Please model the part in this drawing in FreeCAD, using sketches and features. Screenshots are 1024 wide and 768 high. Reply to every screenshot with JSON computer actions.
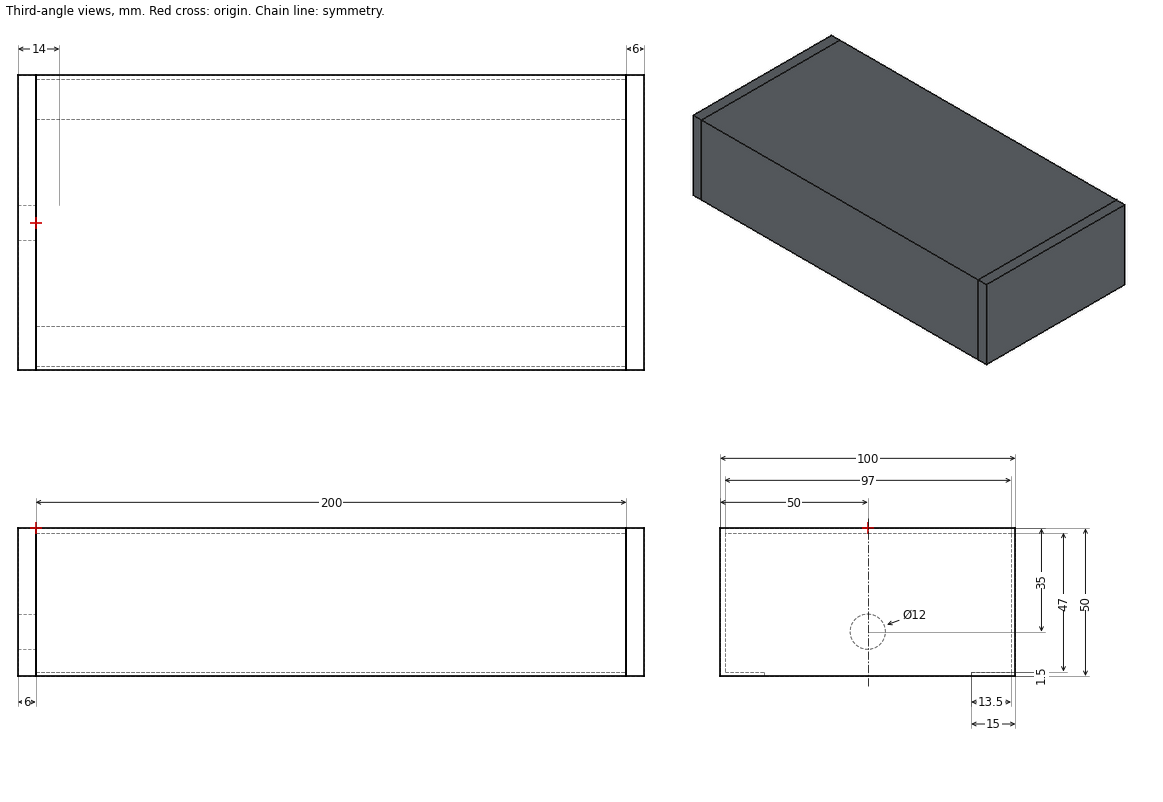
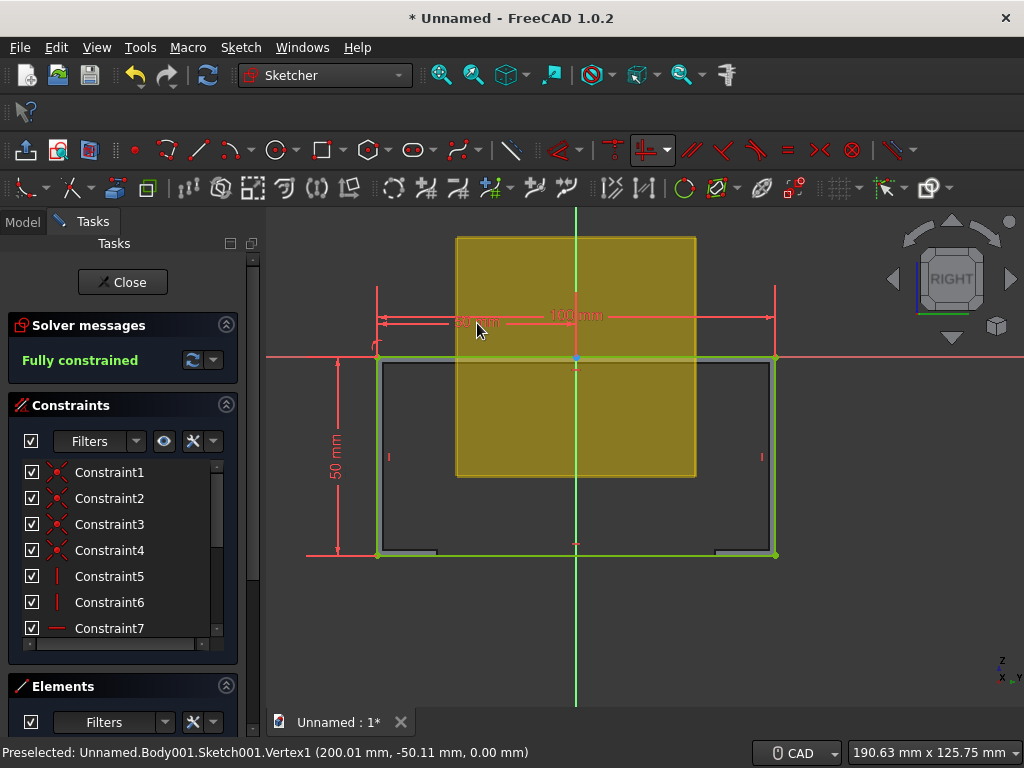
{"action": "left_click", "coordinate": [123, 282]}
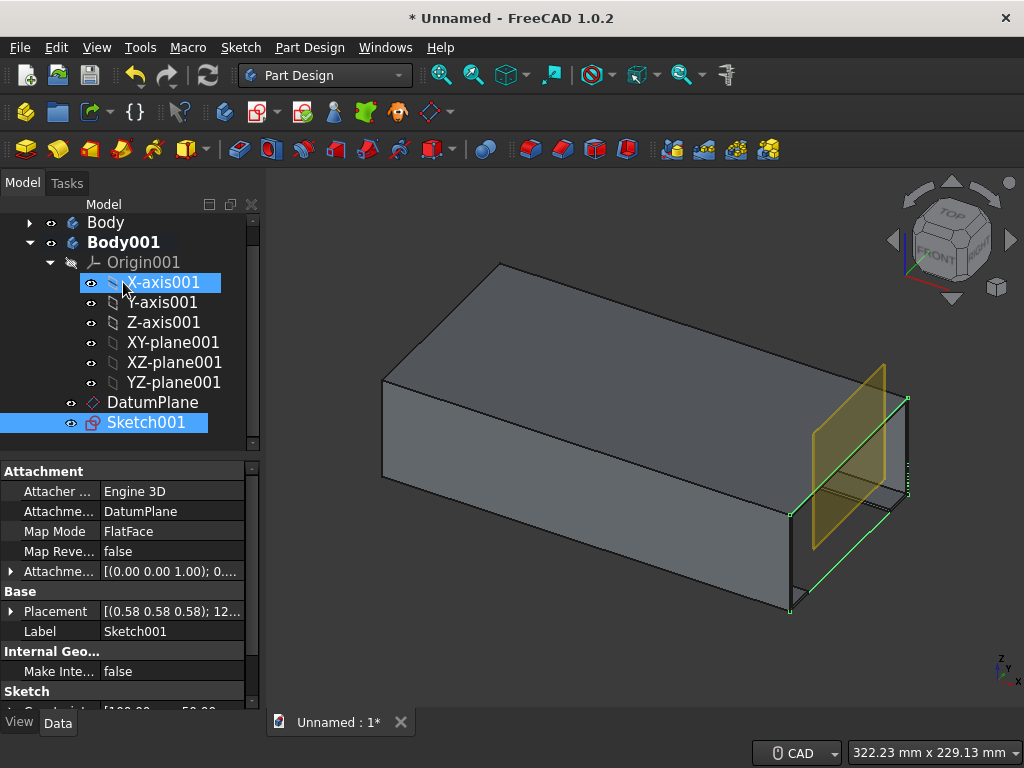
{"action": "left_click", "coordinate": [26, 150]}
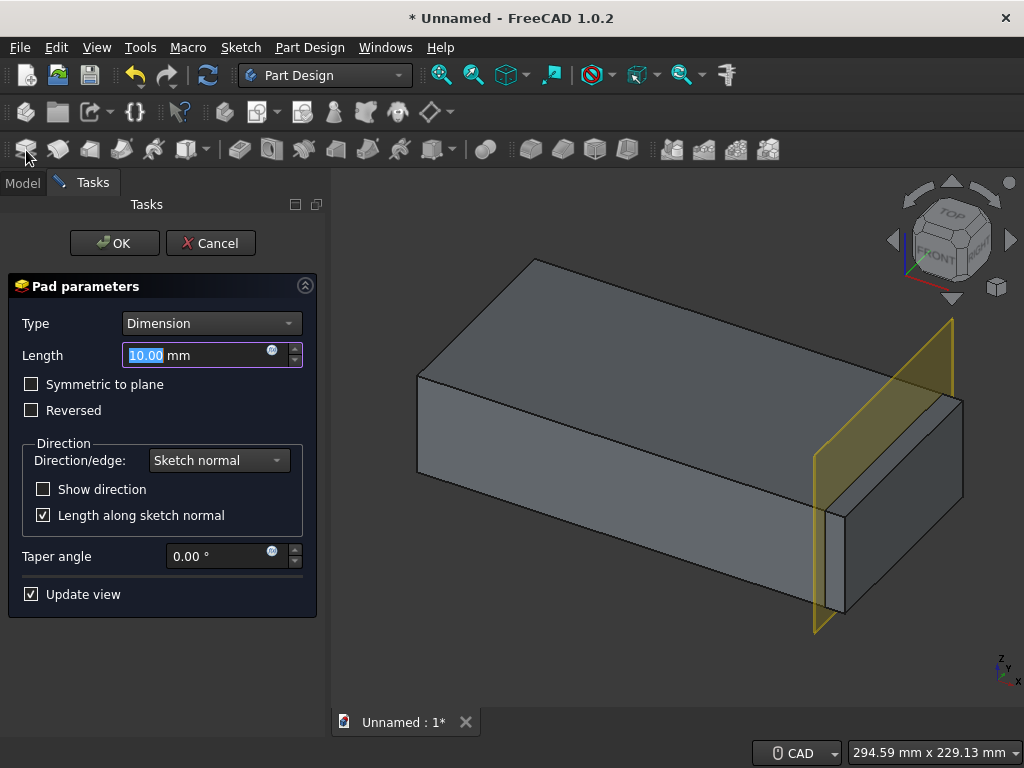
{"action": "type", "text": "6"}
{"action": "key", "text": "Tab"}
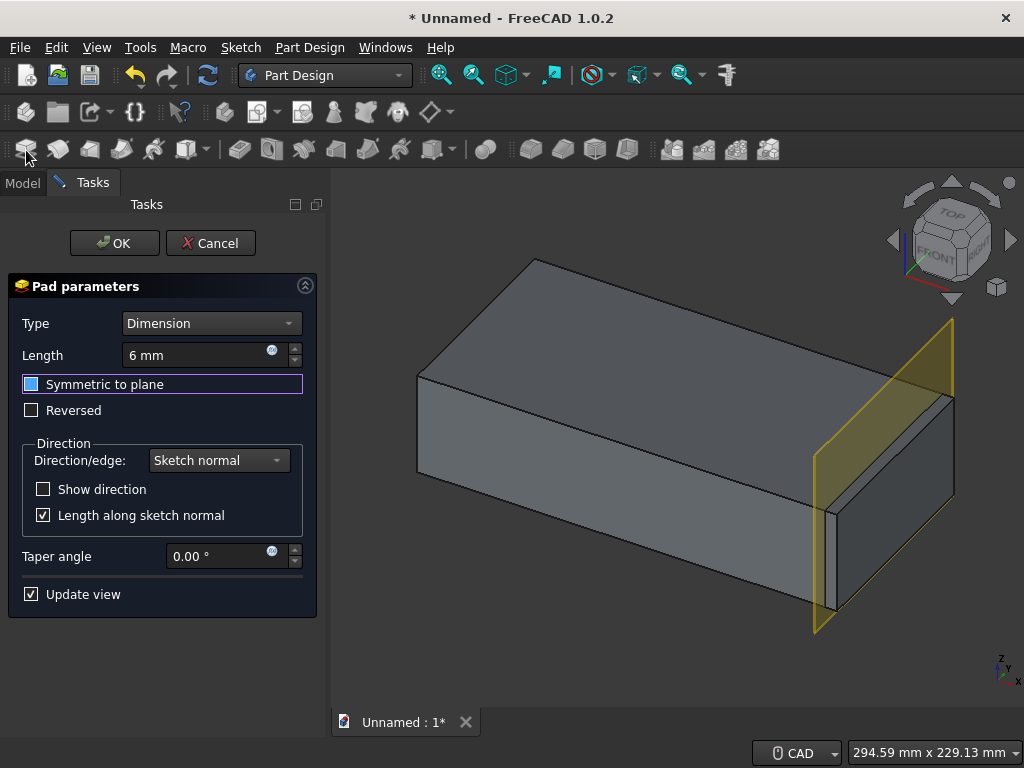
{"action": "left_click", "coordinate": [115, 243]}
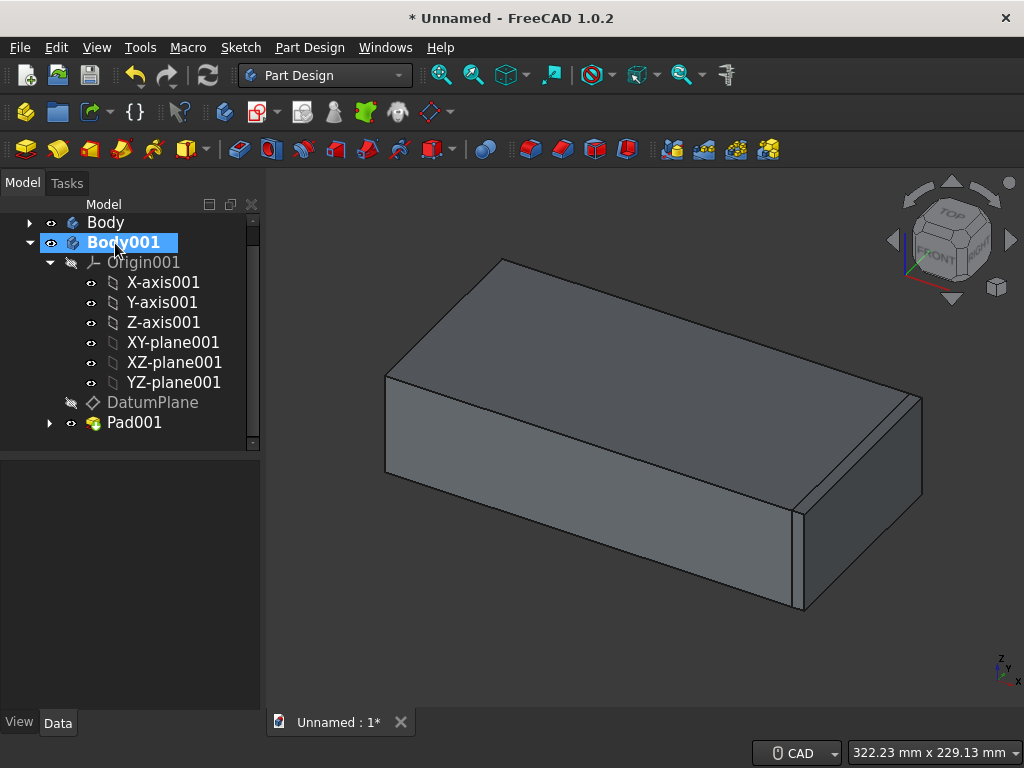
{"action": "left_click", "coordinate": [442, 76]}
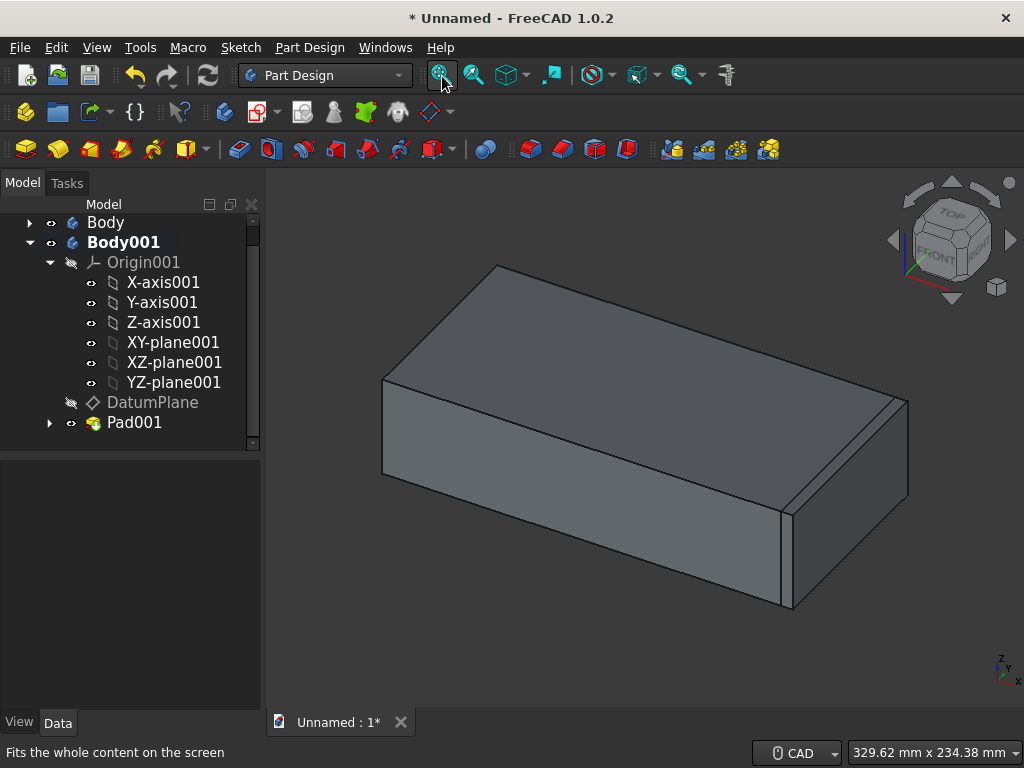
{"action": "left_click", "coordinate": [226, 112]}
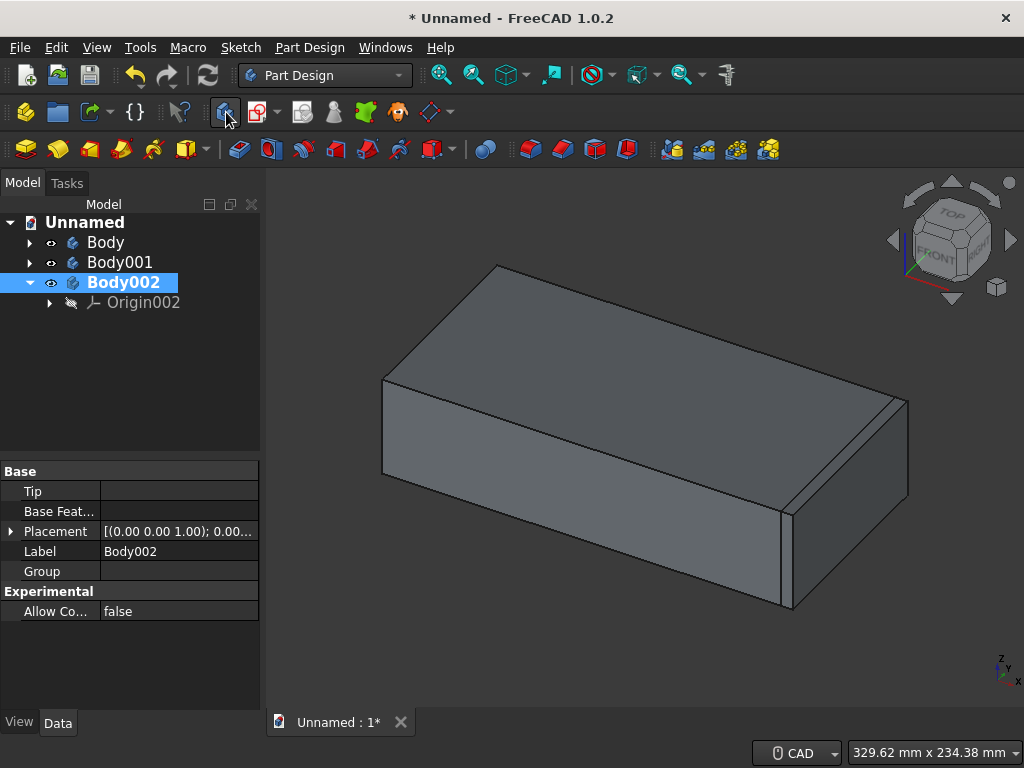
{"action": "left_click", "coordinate": [306, 667]}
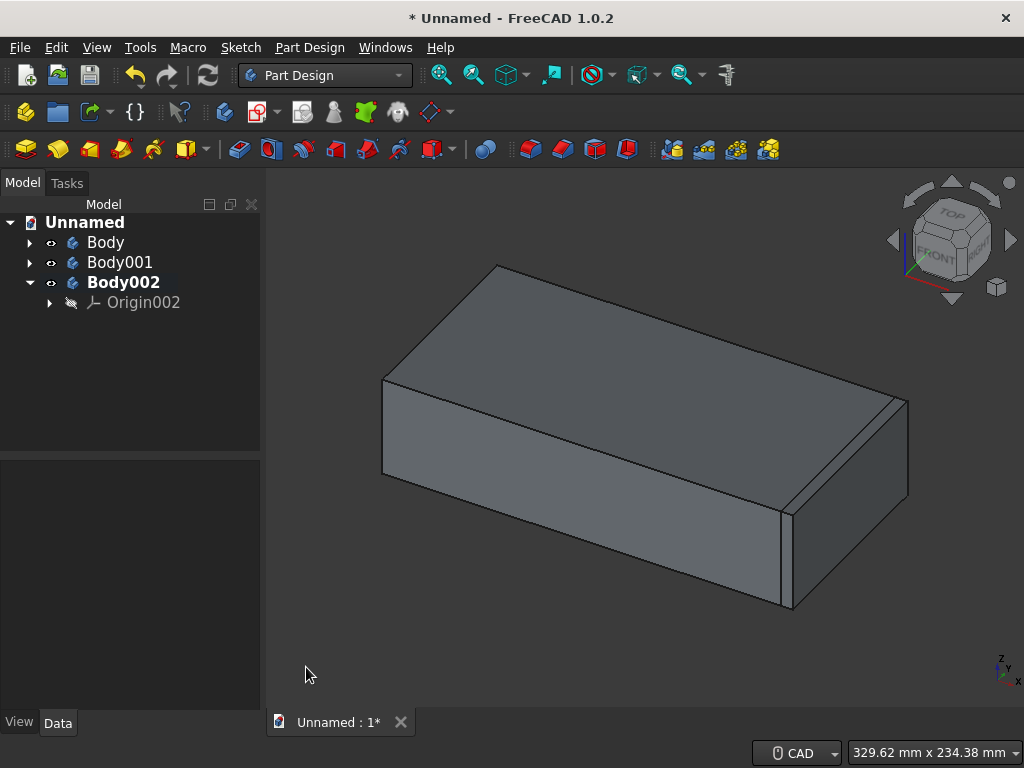
{"action": "left_click", "coordinate": [258, 112]}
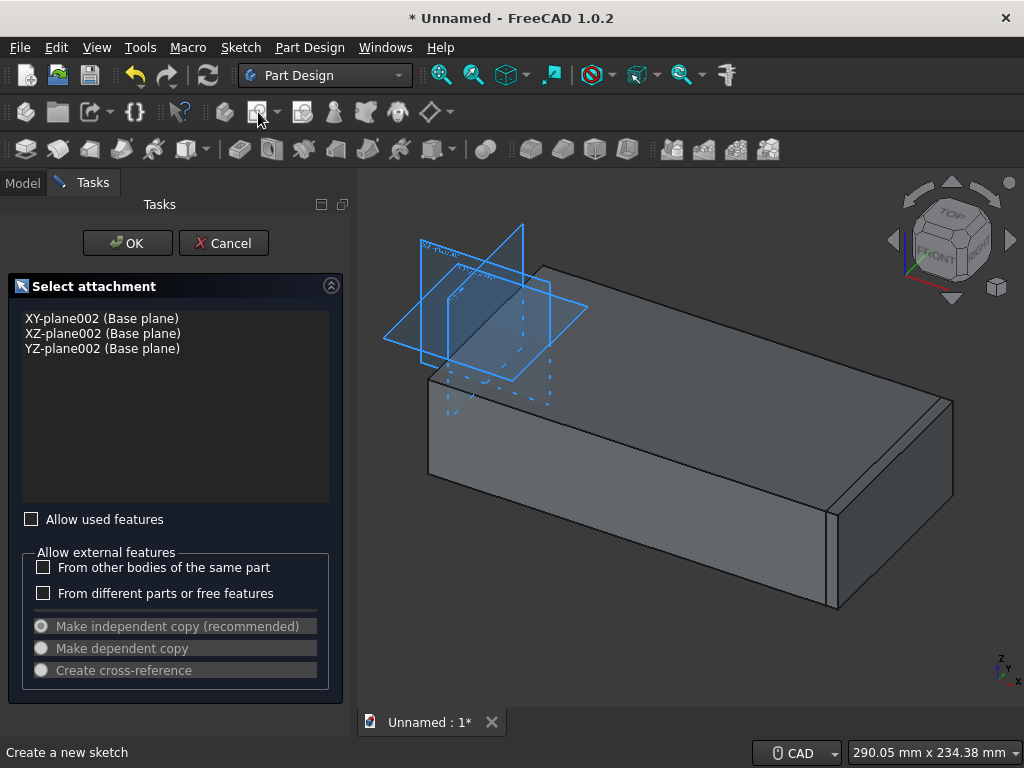
{"action": "left_click", "coordinate": [82, 348]}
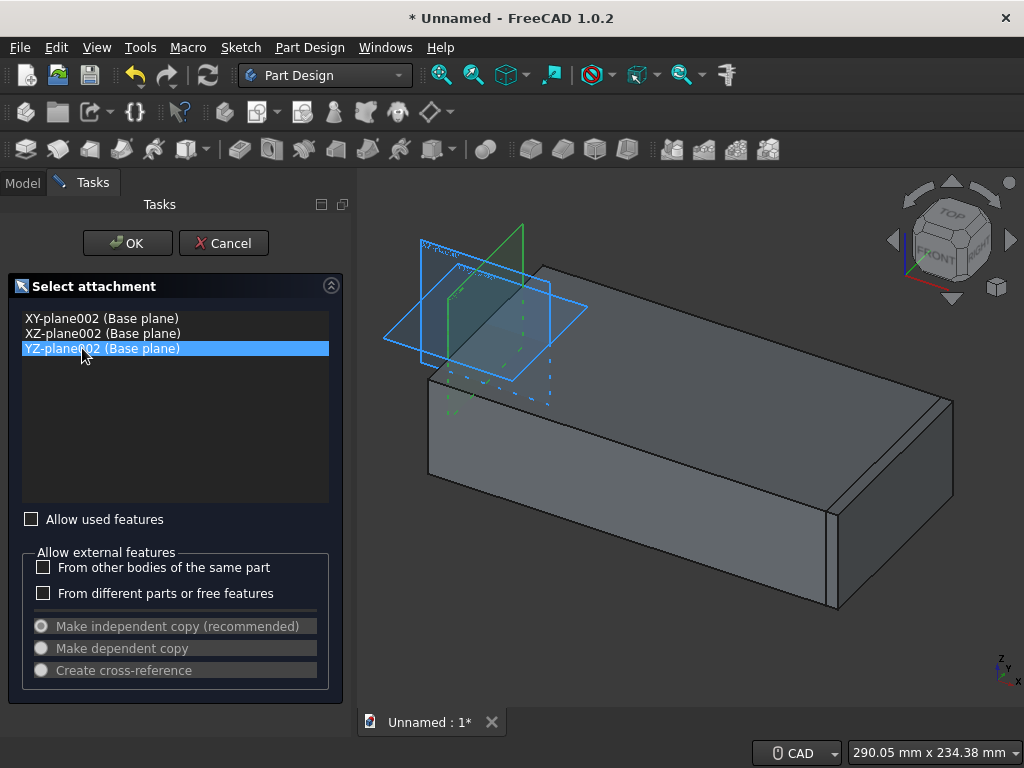
{"action": "left_click", "coordinate": [128, 243]}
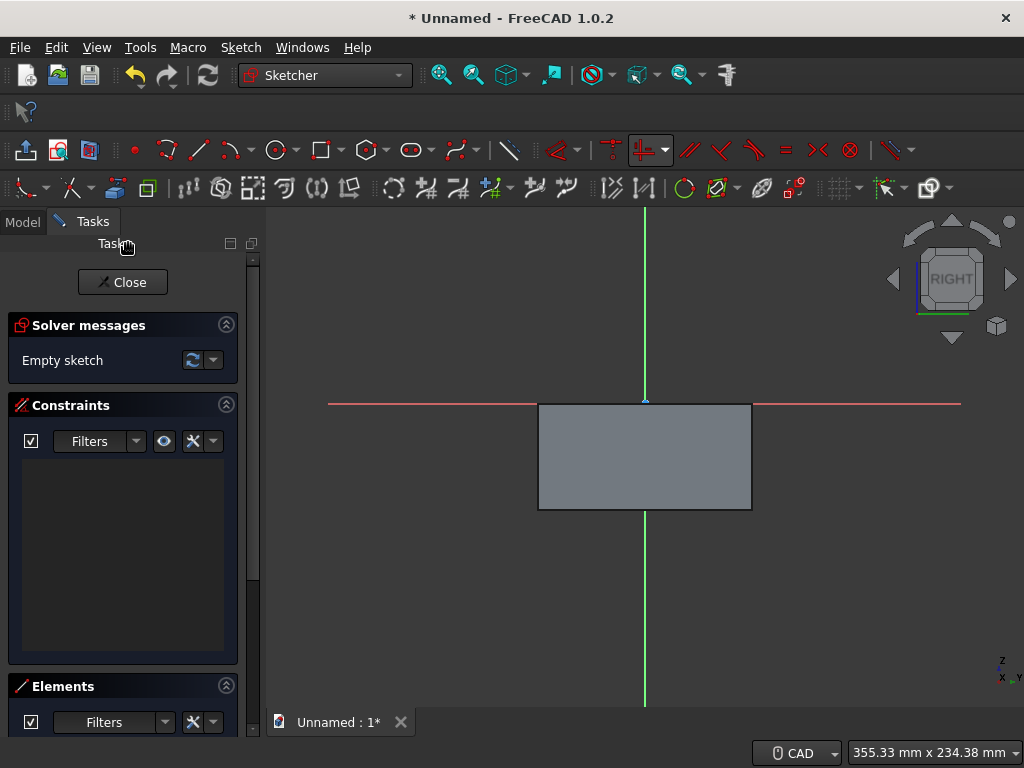
{"action": "scroll", "coordinate": [728, 457], "scroll_direction": "up", "scroll_amount": 3}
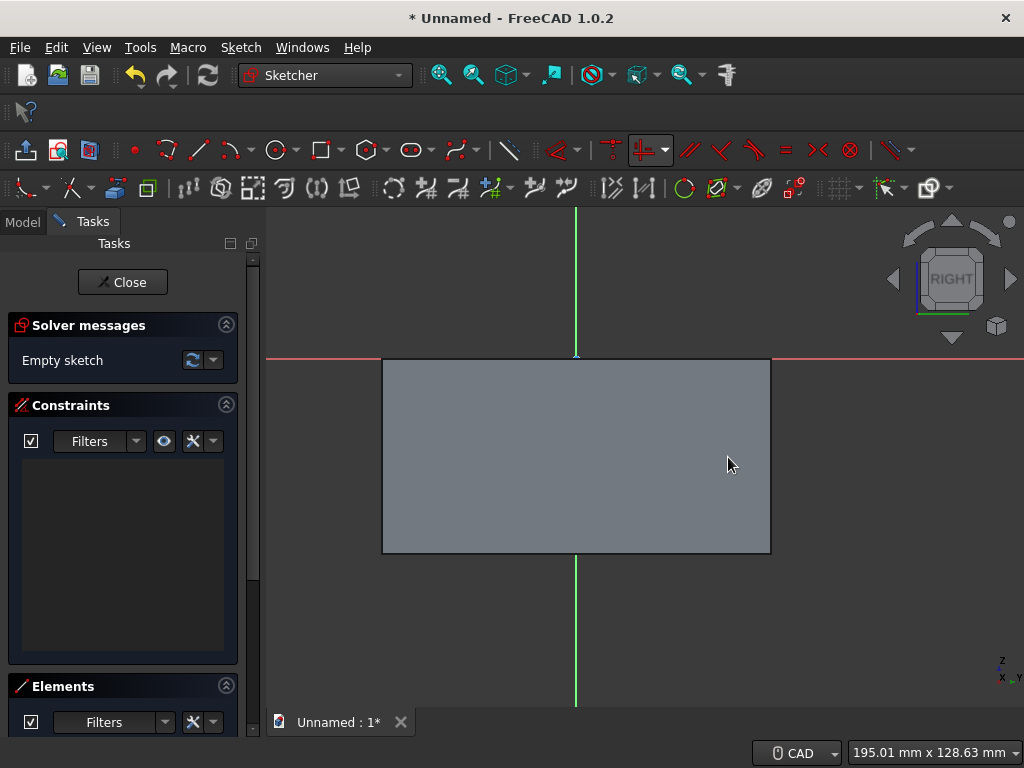
{"action": "left_click", "coordinate": [322, 150]}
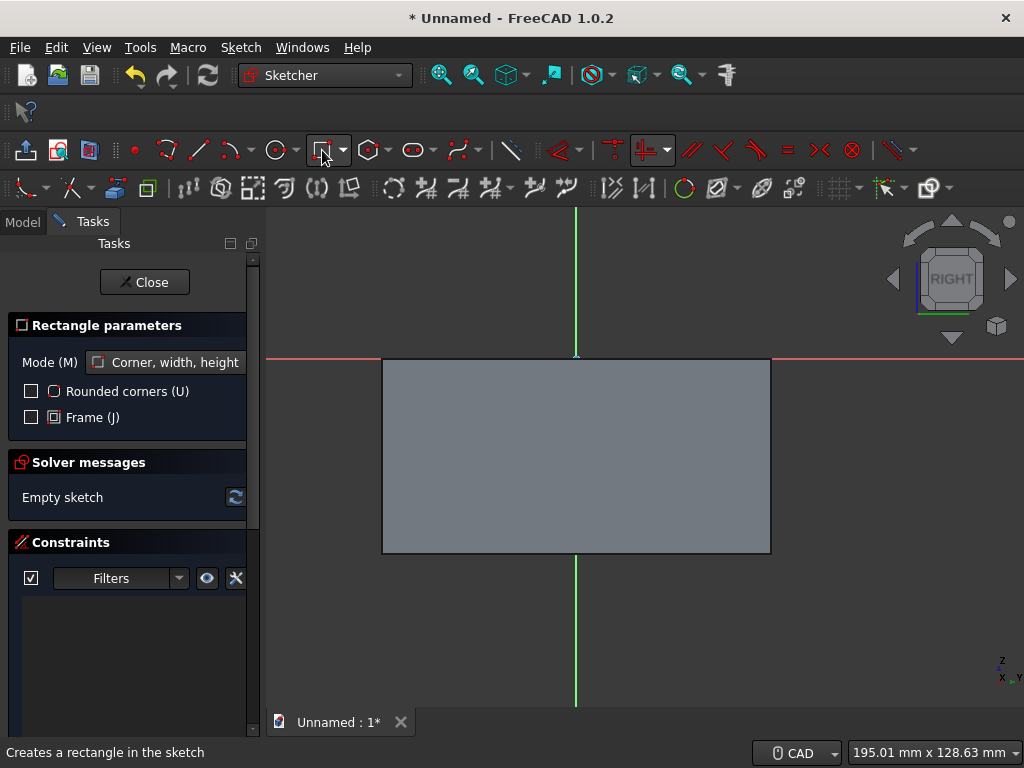
{"action": "left_click", "coordinate": [382, 359]}
{"action": "mouse_move", "coordinate": [771, 554]}